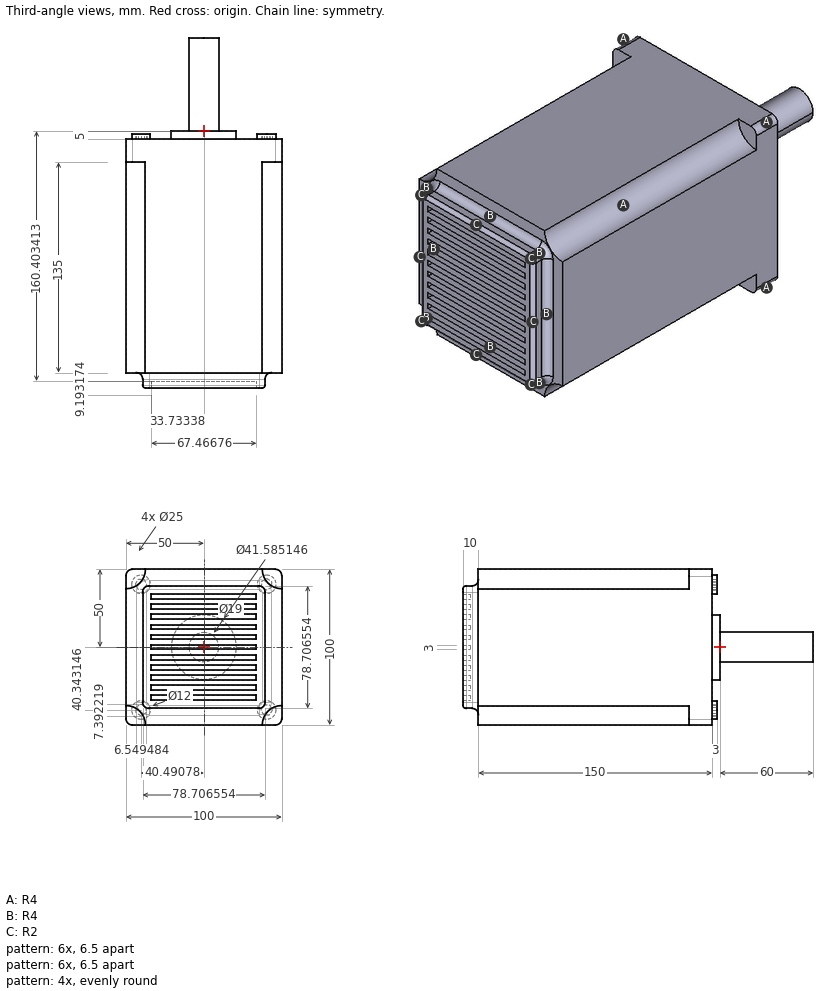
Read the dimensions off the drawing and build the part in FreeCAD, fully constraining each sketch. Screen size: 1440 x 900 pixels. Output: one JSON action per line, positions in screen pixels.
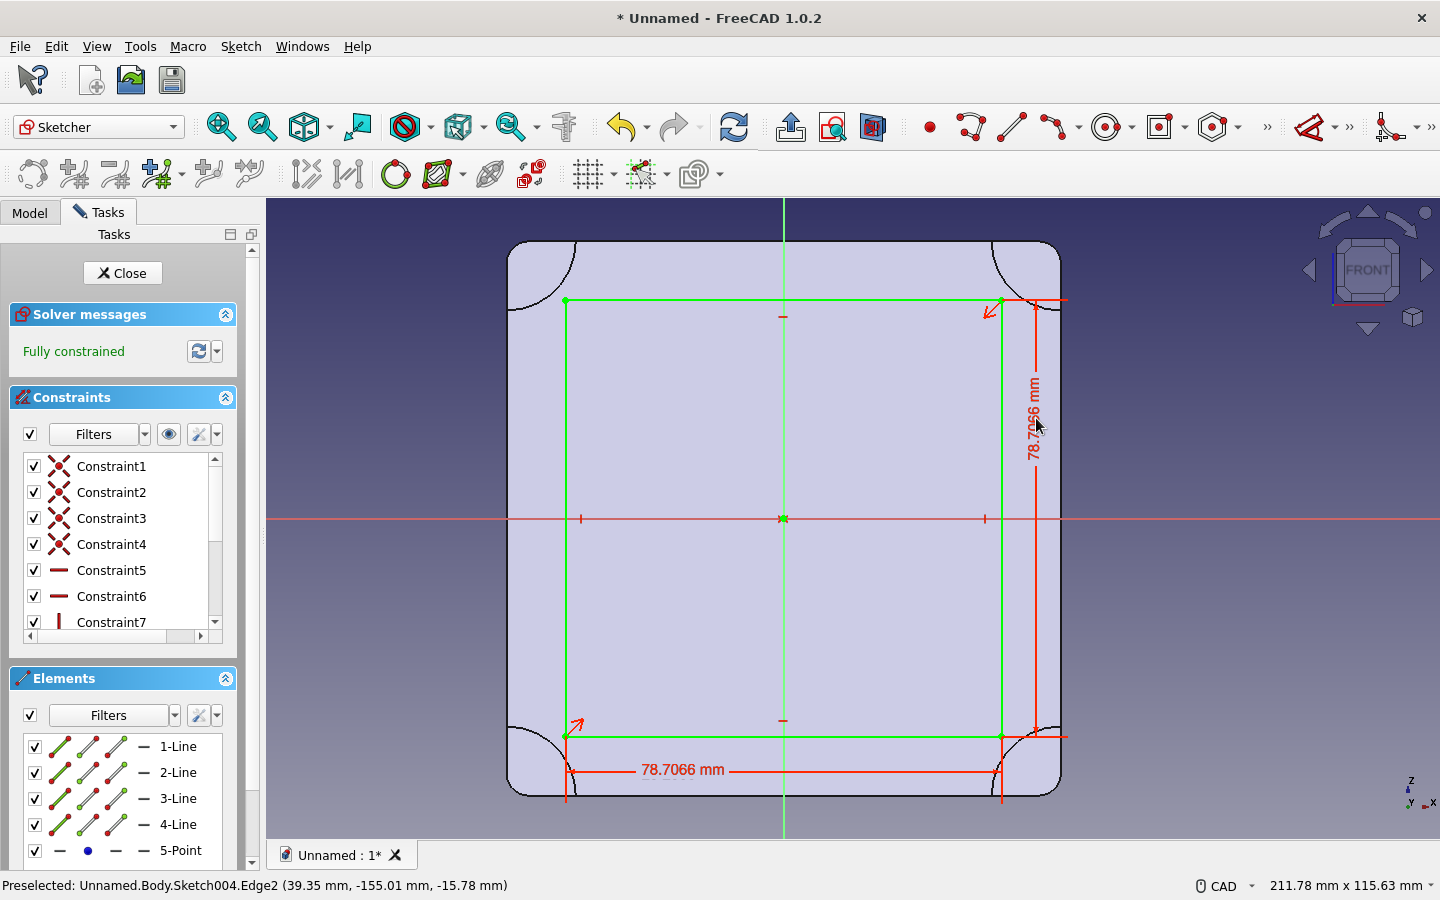
{"action": "left_click", "coordinate": [123, 273]}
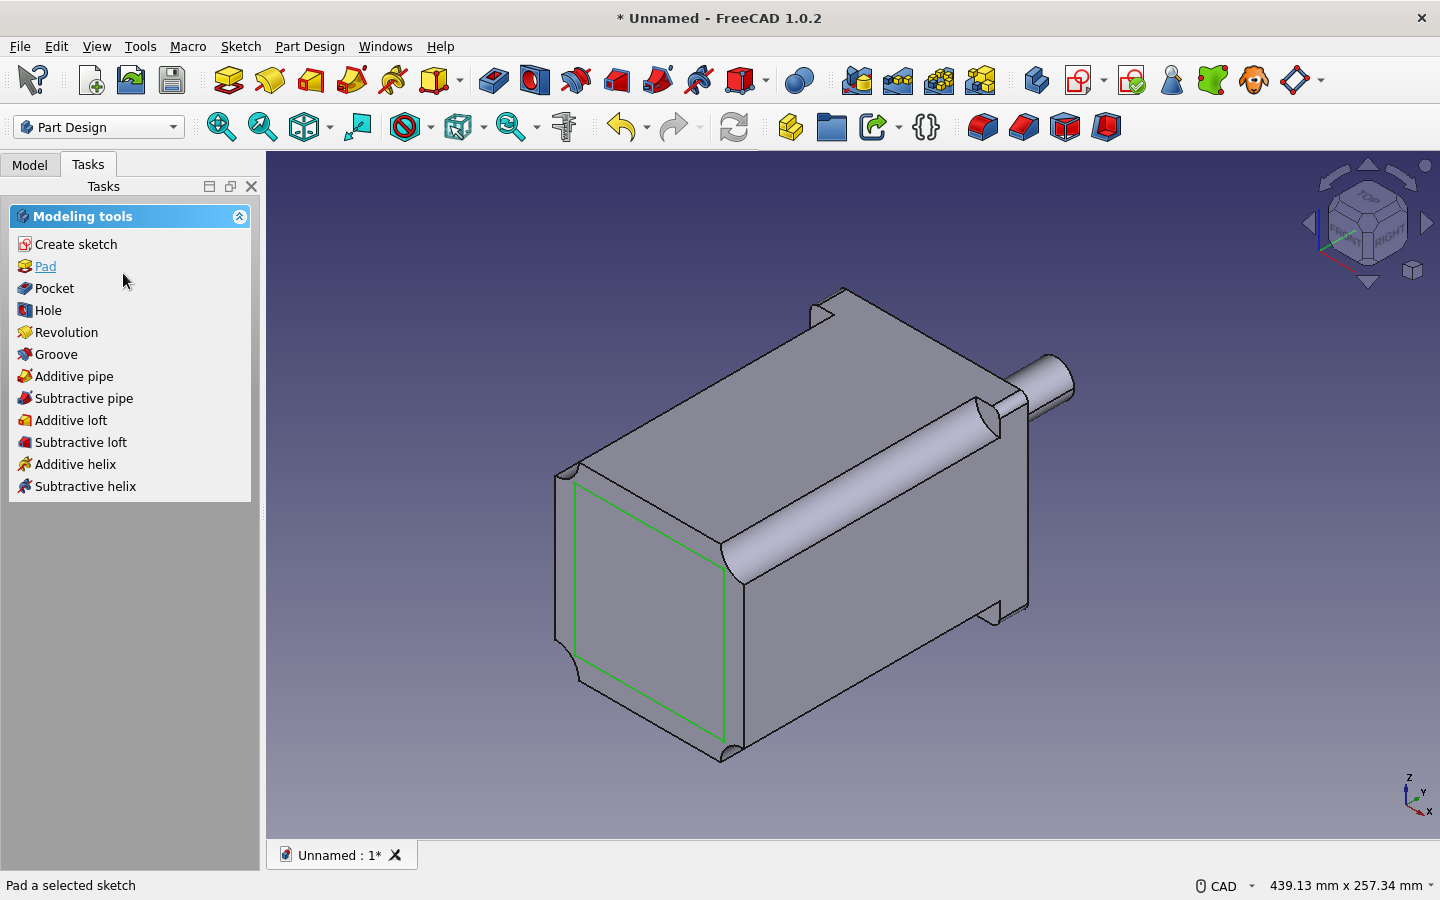
{"action": "left_click", "coordinate": [229, 80]}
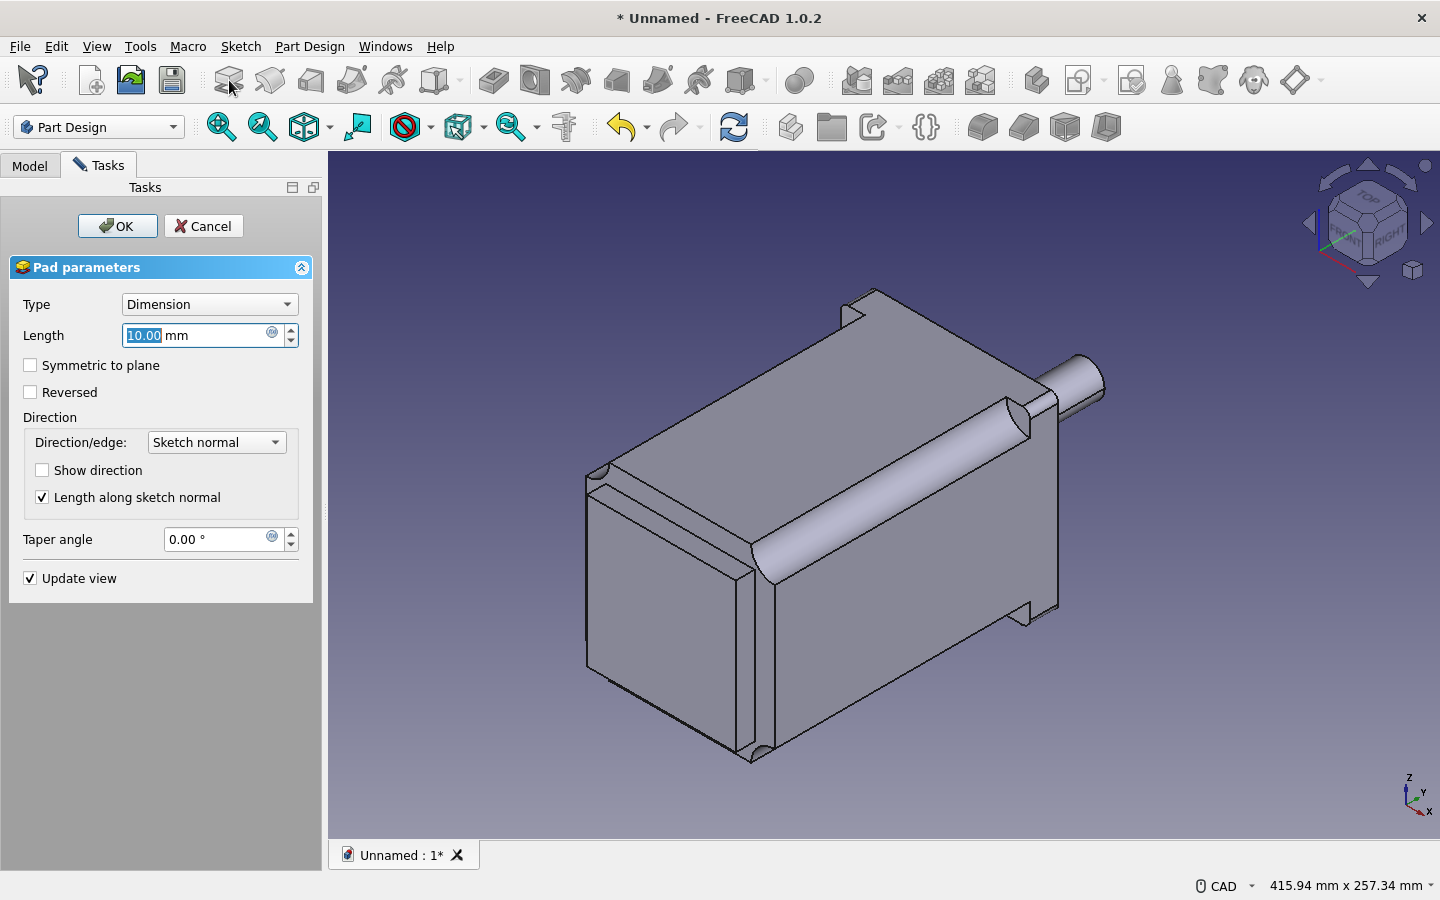
{"action": "type", "text": "10"}
{"action": "key", "text": "Tab"}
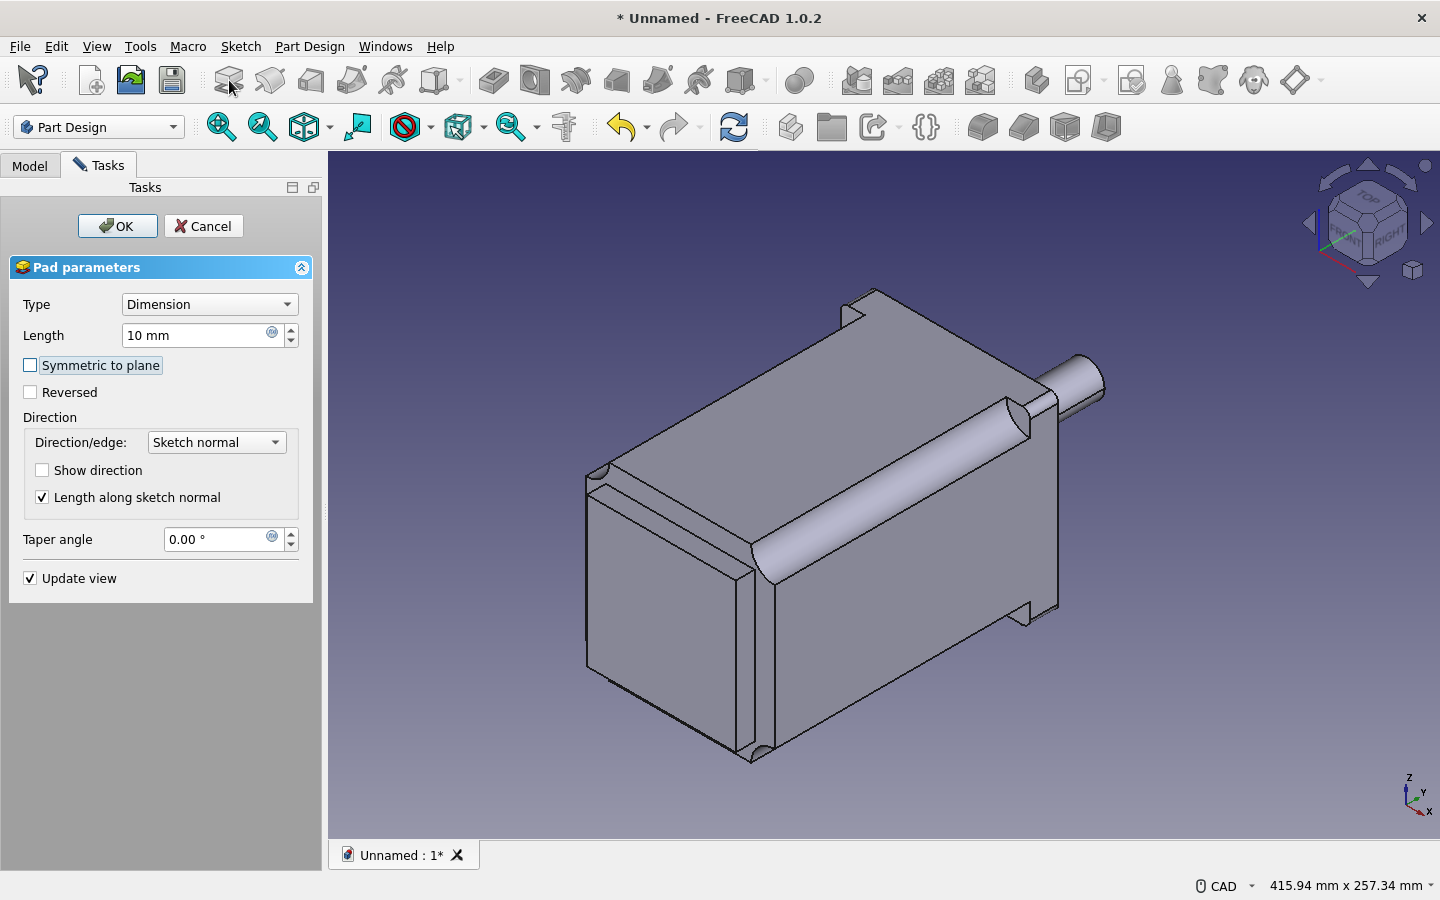
{"action": "left_click", "coordinate": [118, 226]}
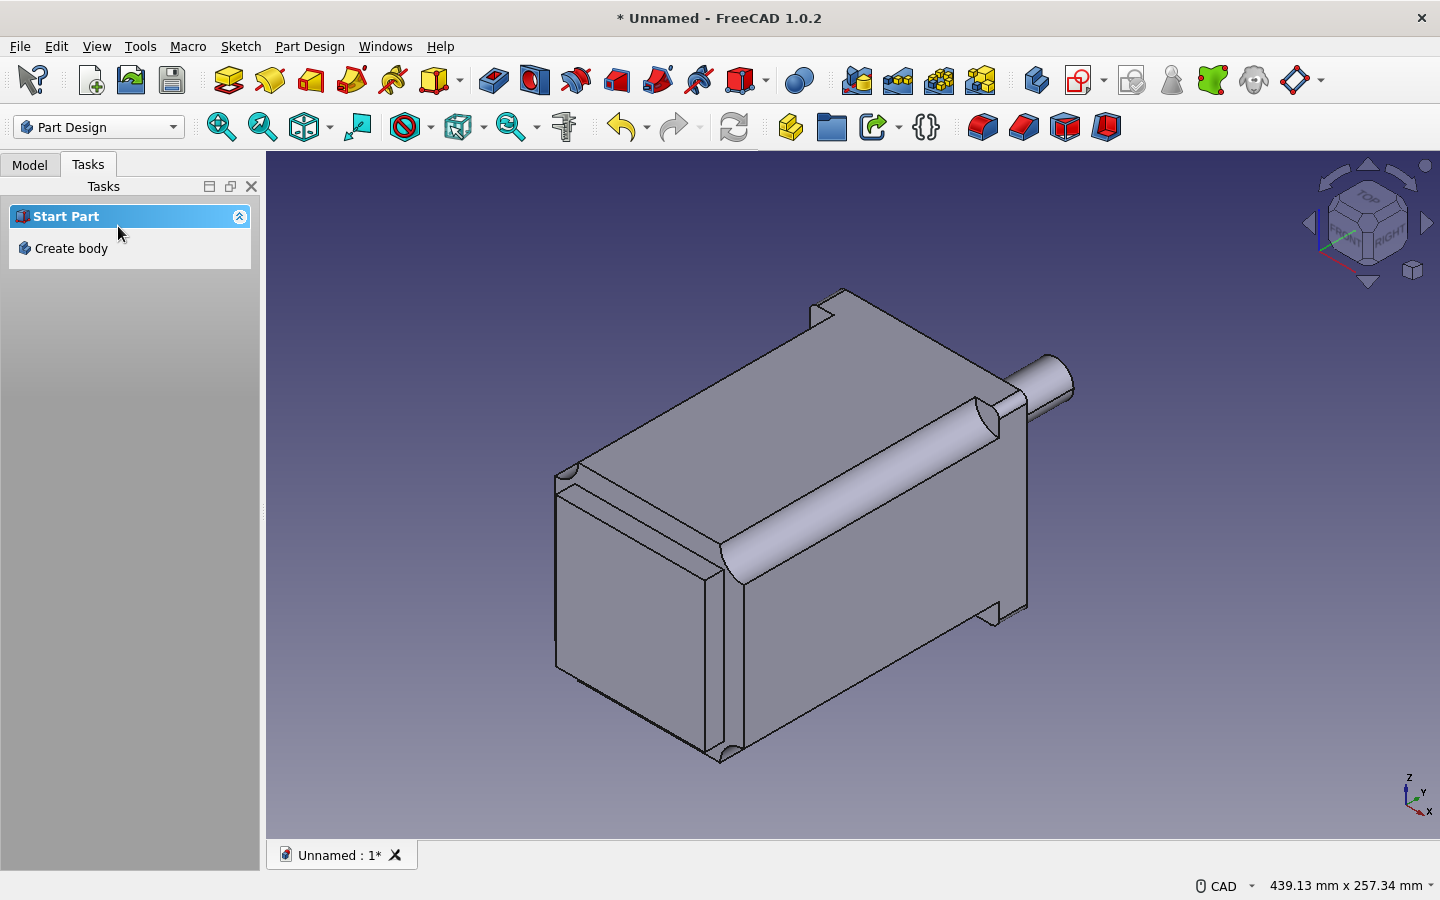
{"action": "left_click", "coordinate": [714, 574]}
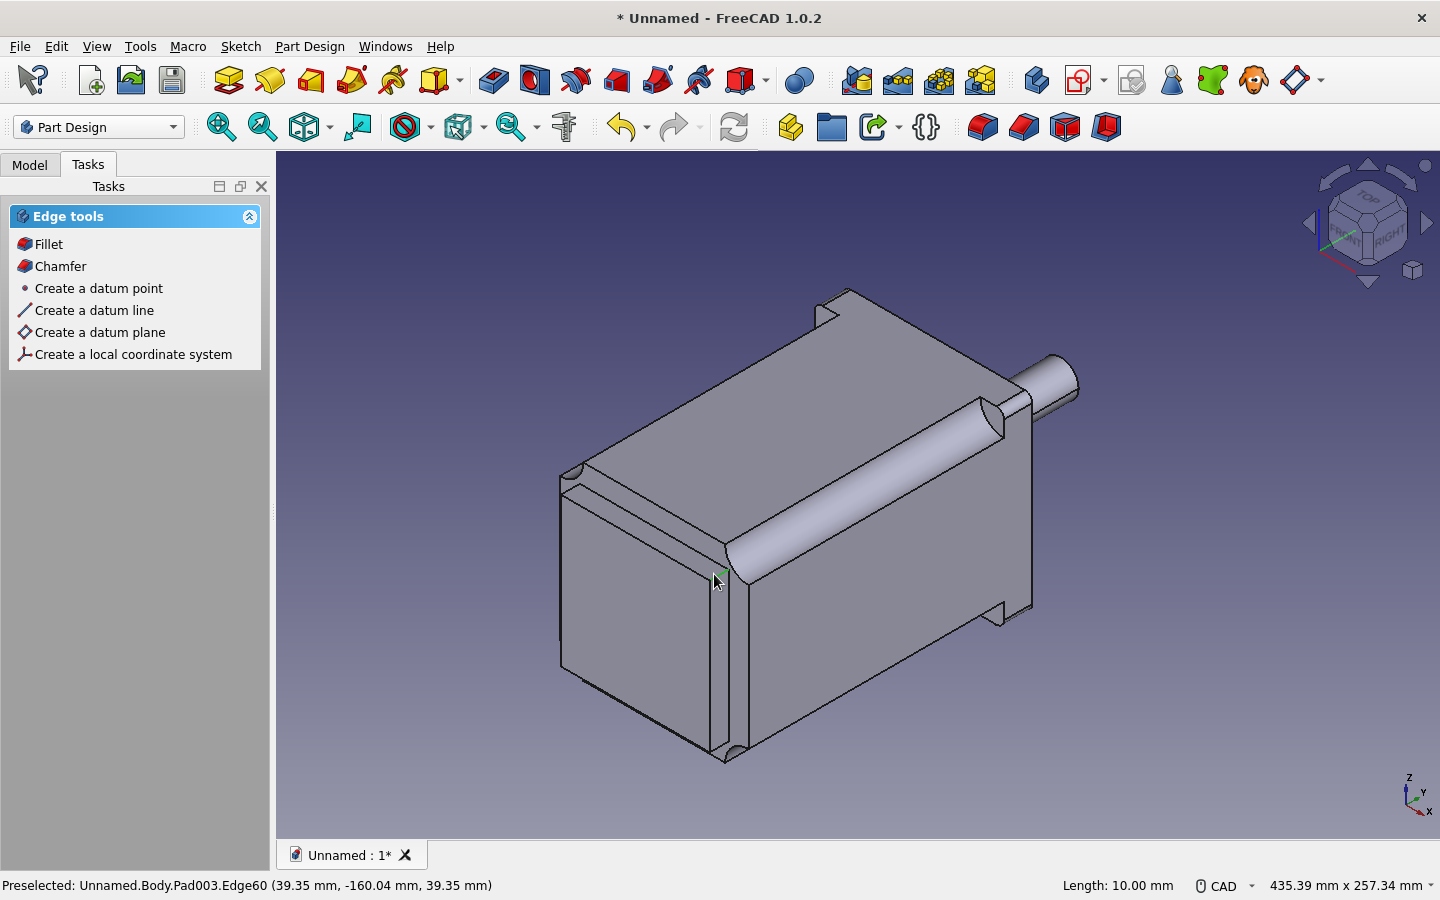
{"action": "key", "text": "2"}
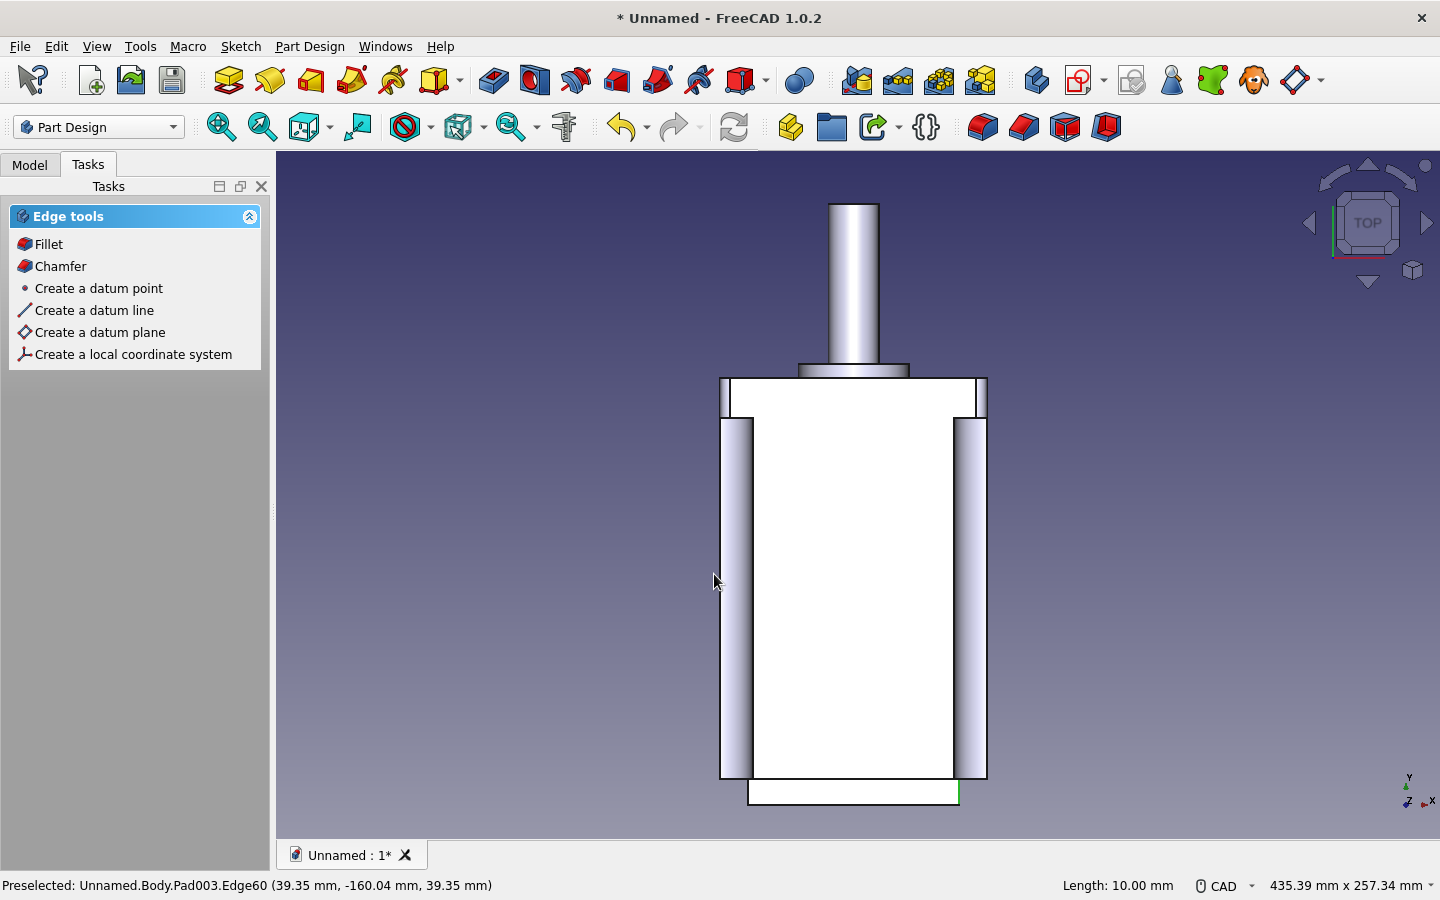
{"action": "left_click", "coordinate": [748, 791], "text": "ctrl"}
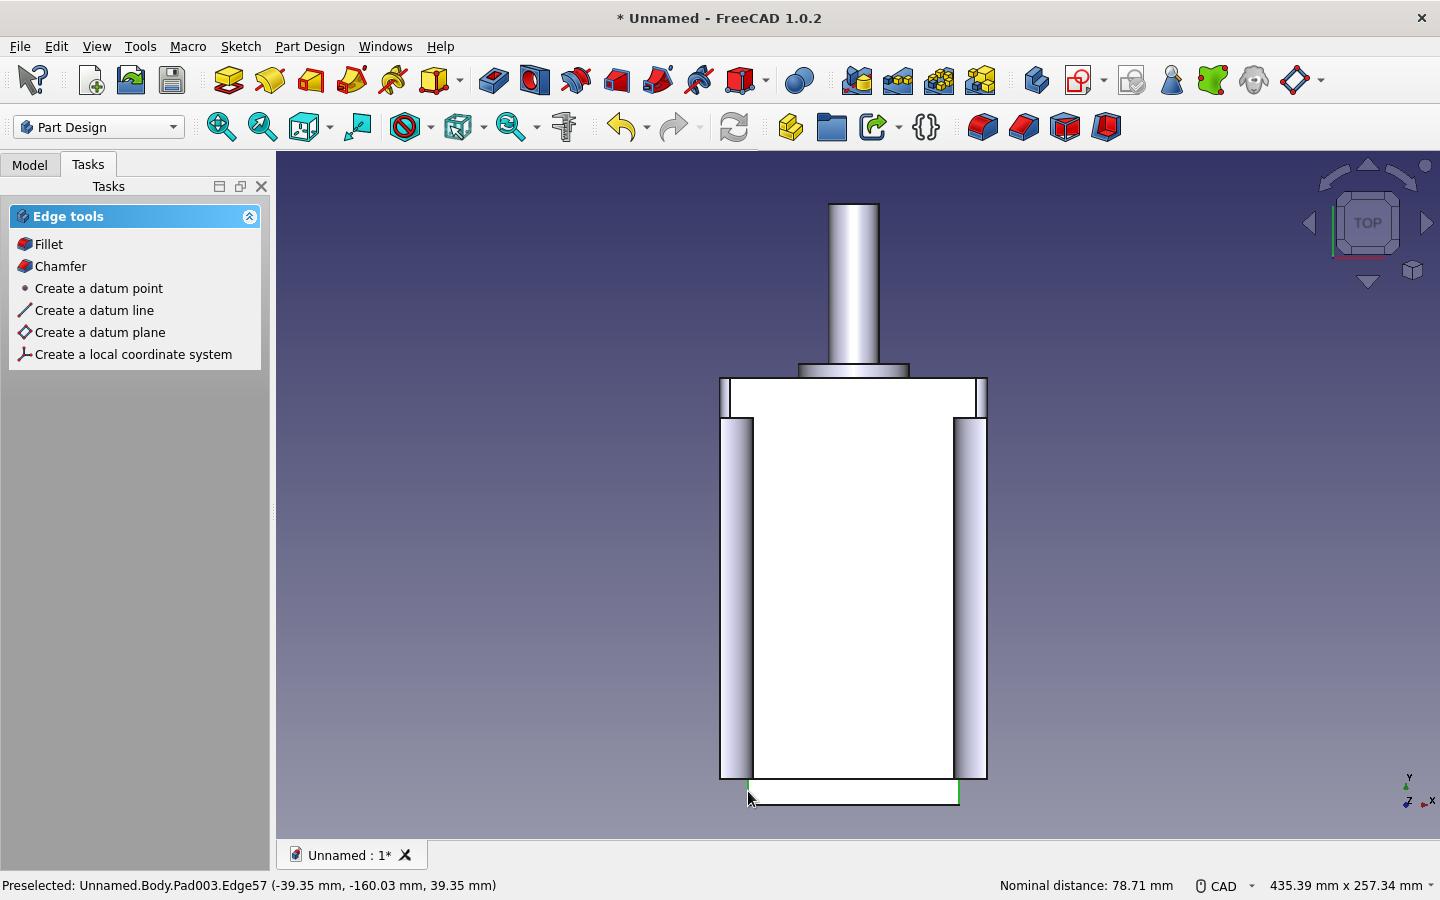
{"action": "key", "text": "0"}